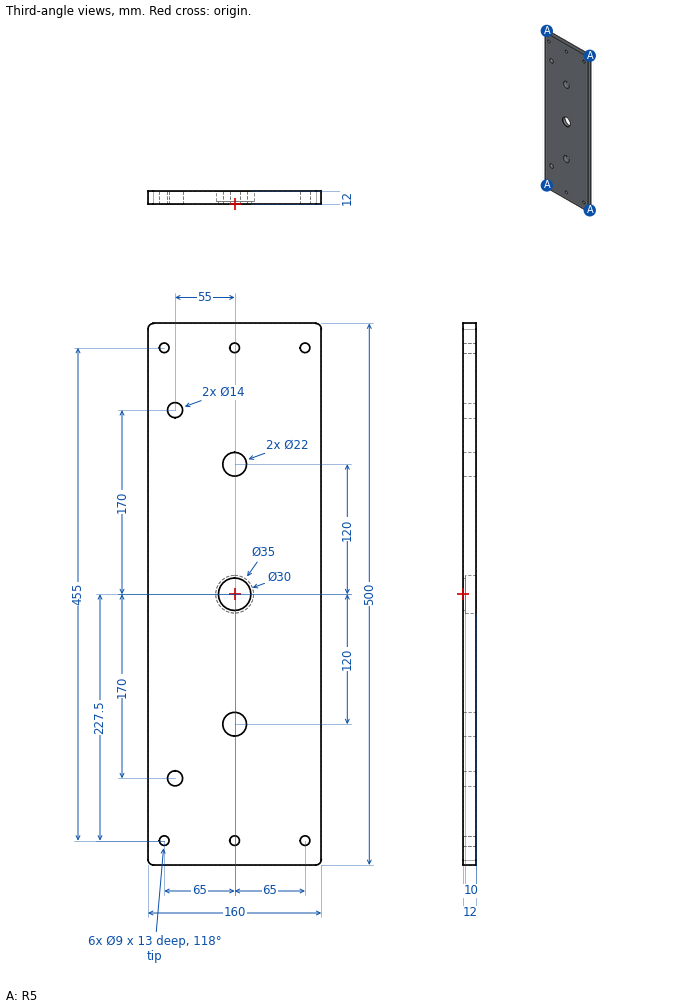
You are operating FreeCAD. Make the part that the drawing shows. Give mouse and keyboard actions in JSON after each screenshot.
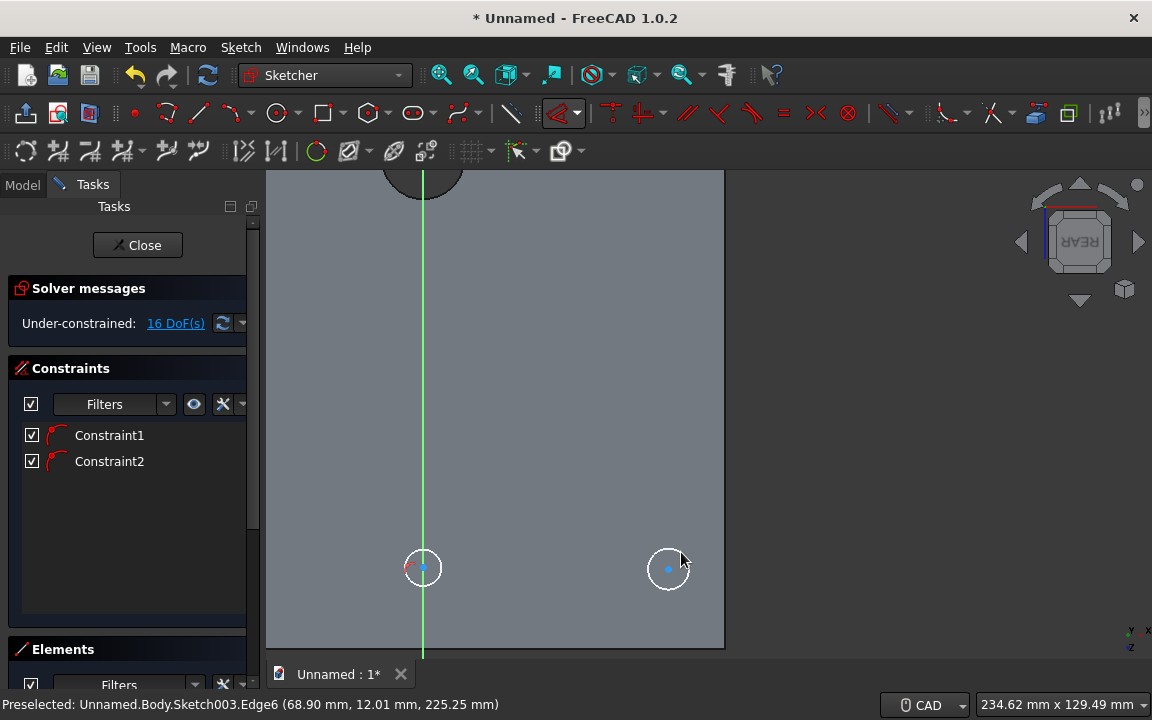
{"action": "scroll", "coordinate": [684, 555], "scroll_direction": "down", "scroll_amount": 9}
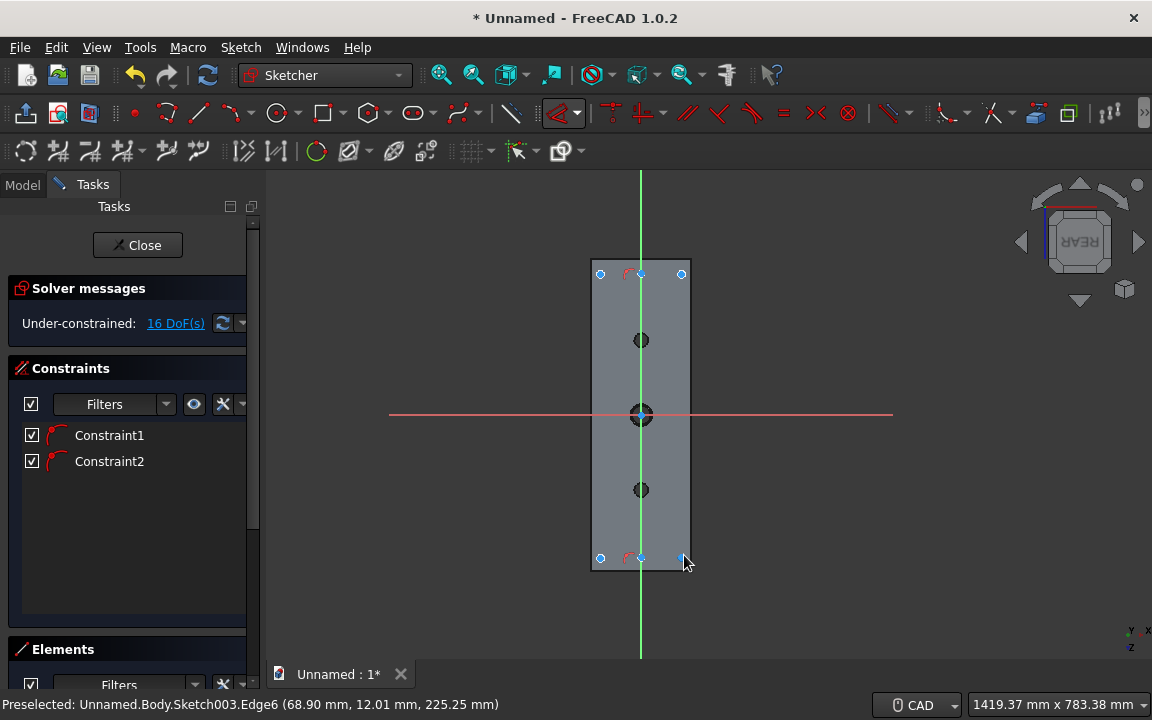
{"action": "scroll", "coordinate": [603, 272], "scroll_direction": "up", "scroll_amount": 7}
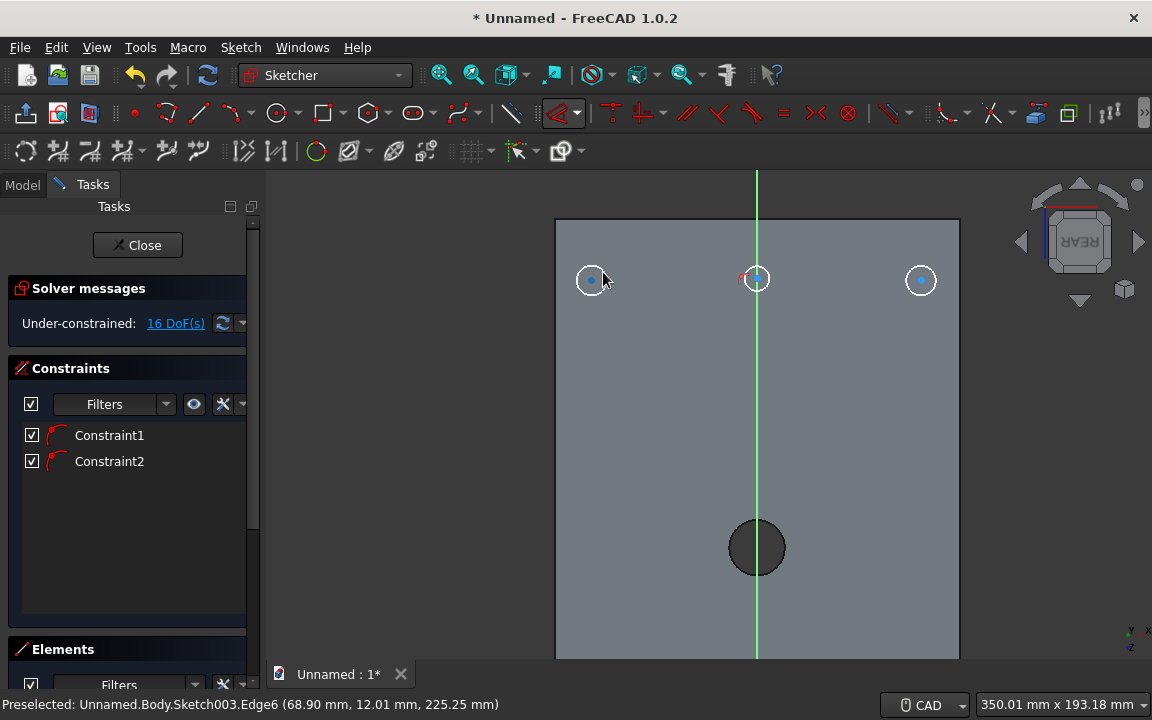
{"action": "left_click", "coordinate": [602, 270]}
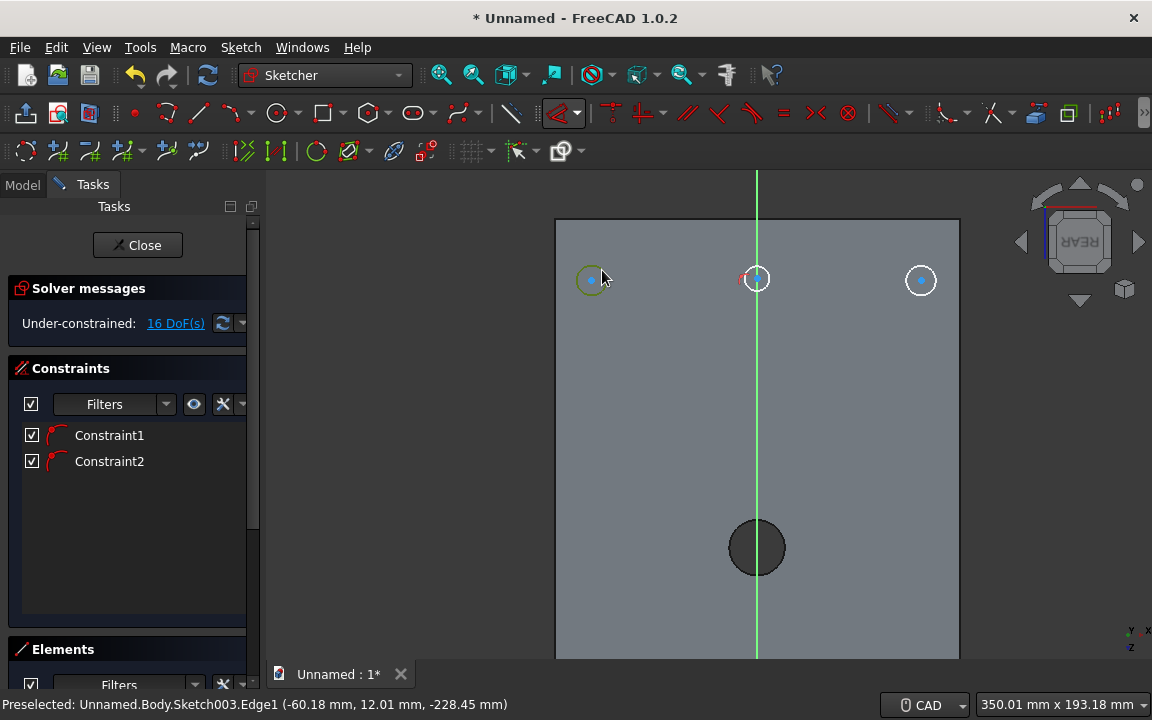
{"action": "left_click", "coordinate": [757, 266]}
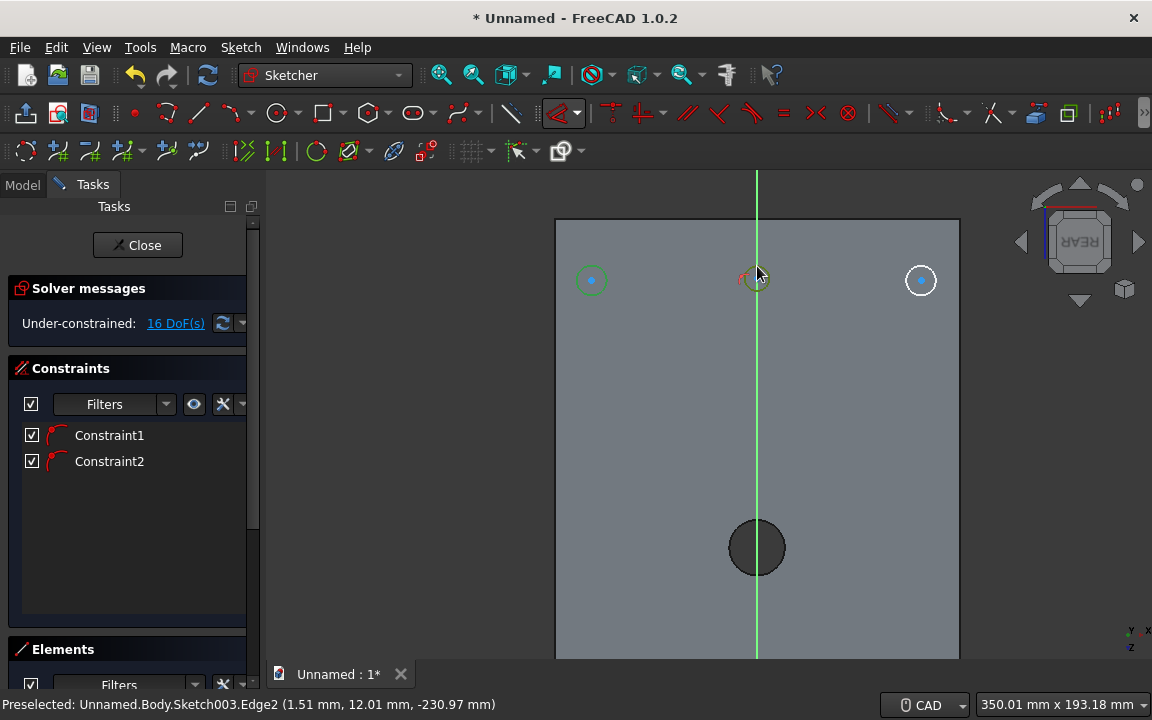
{"action": "left_click", "coordinate": [931, 270]}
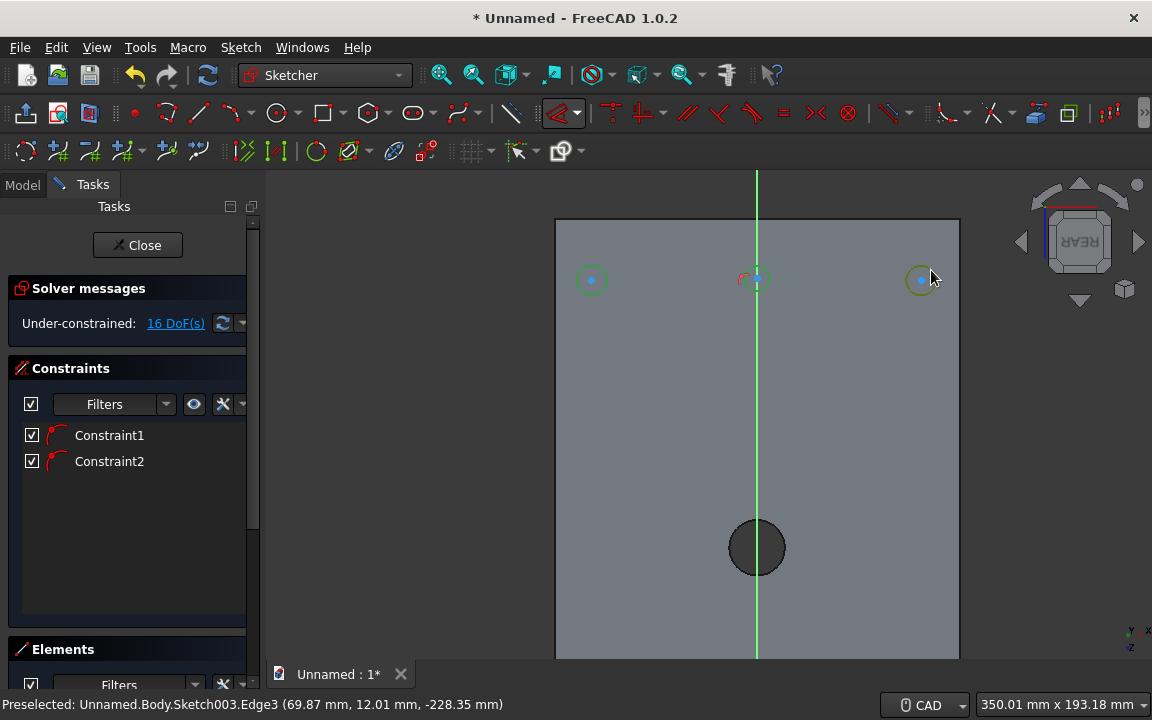
{"action": "scroll", "coordinate": [602, 271], "scroll_direction": "down", "scroll_amount": 7}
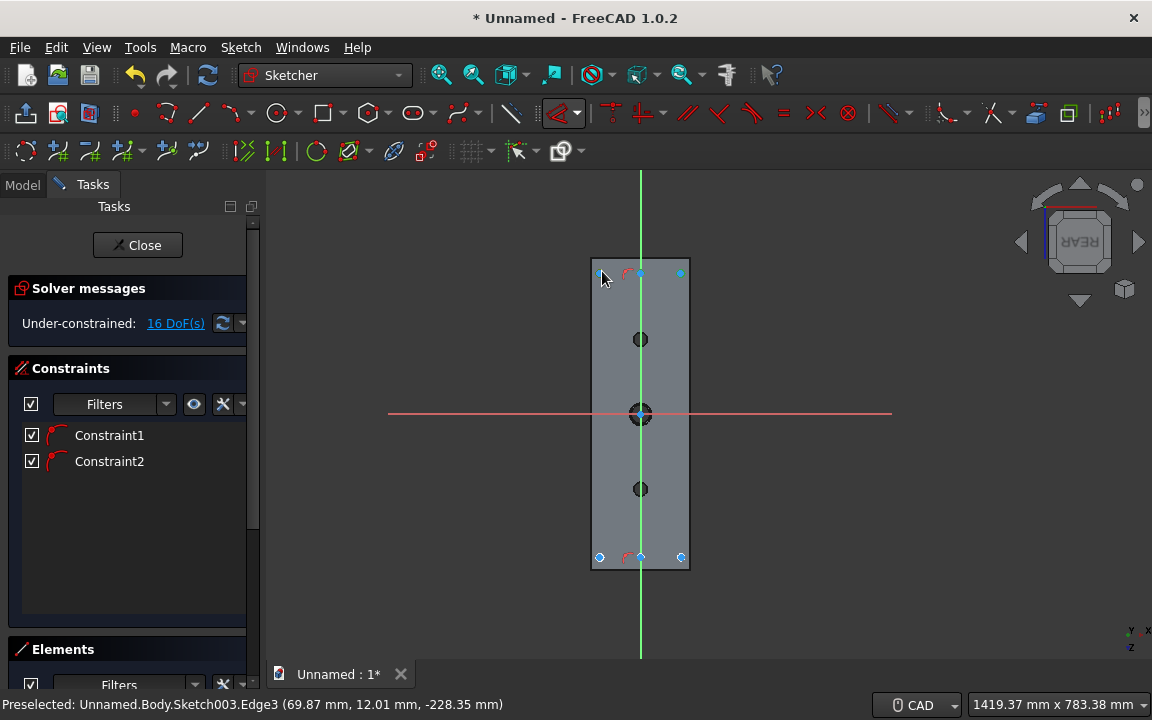
{"action": "scroll", "coordinate": [603, 555], "scroll_direction": "up", "scroll_amount": 7}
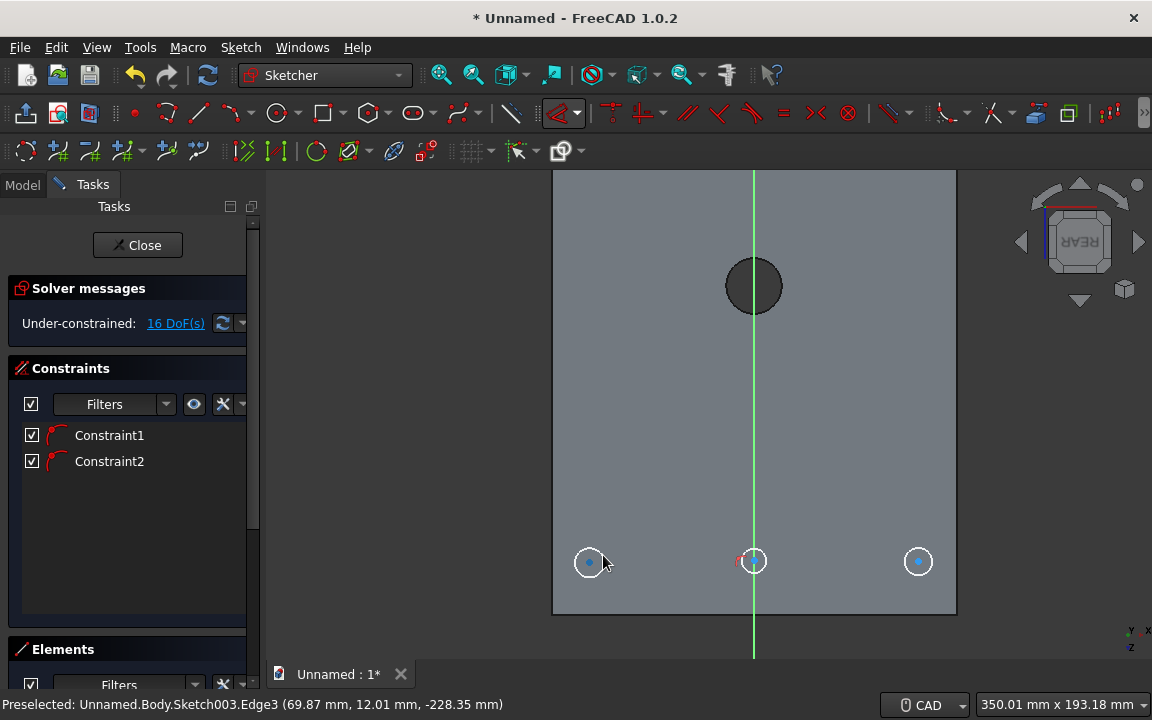
{"action": "left_click", "coordinate": [600, 553]}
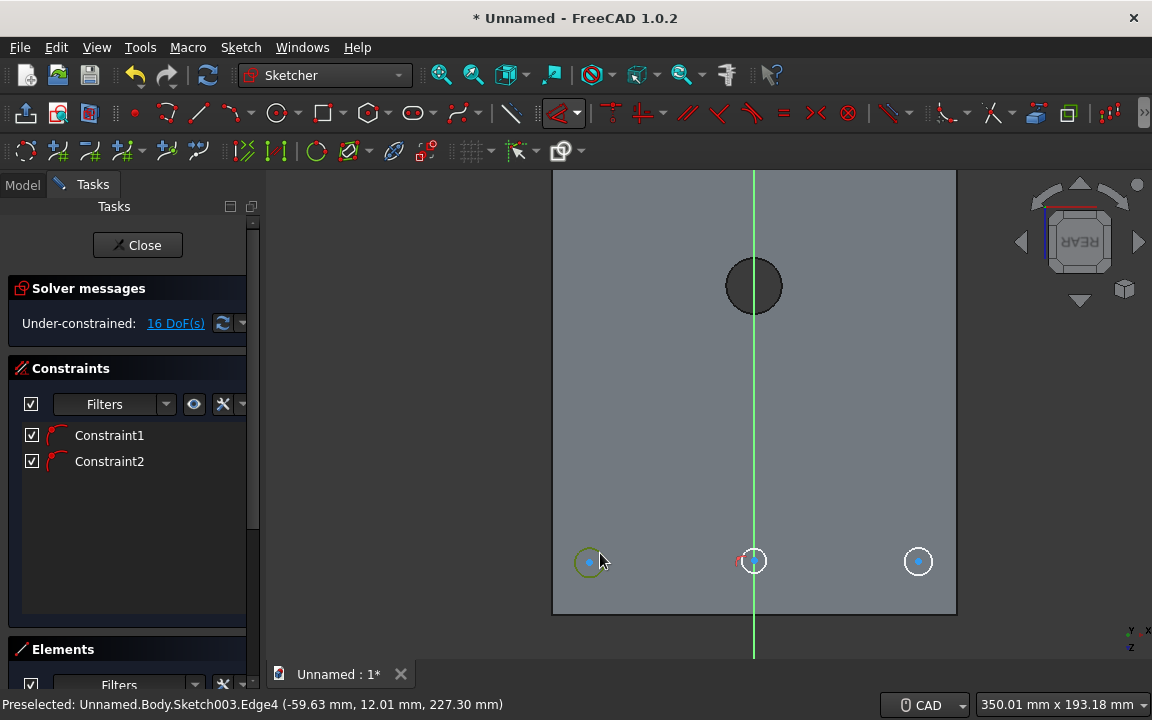
{"action": "left_click", "coordinate": [754, 549]}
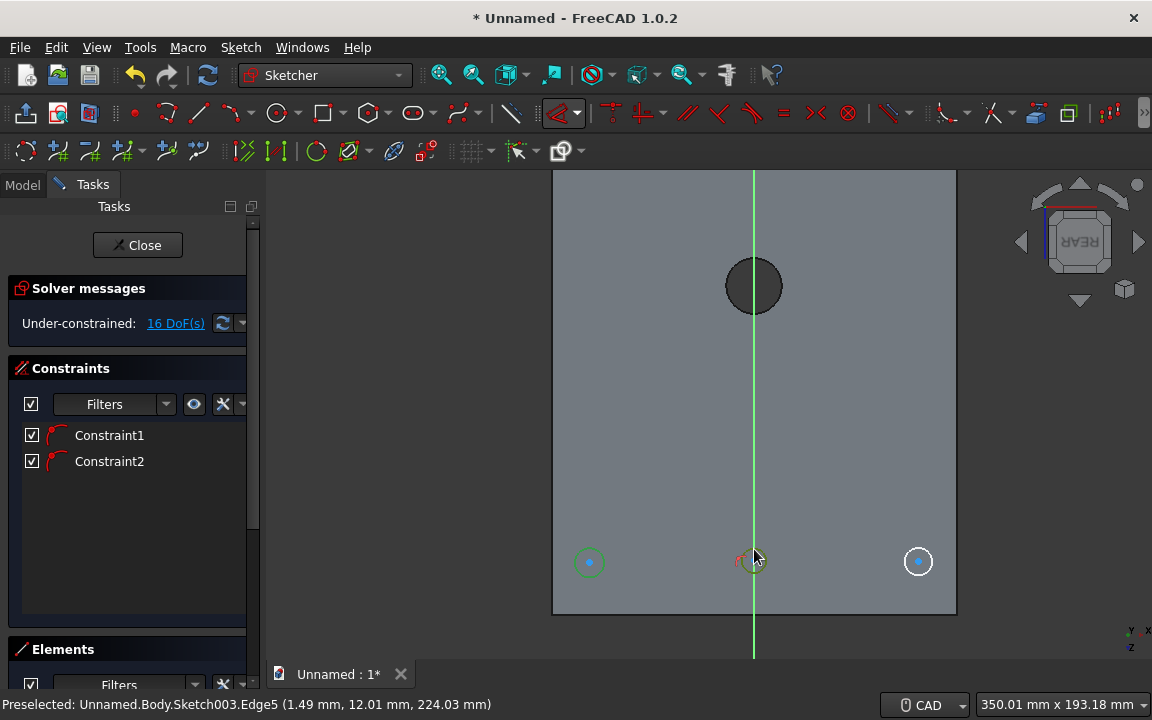
{"action": "left_click", "coordinate": [928, 552]}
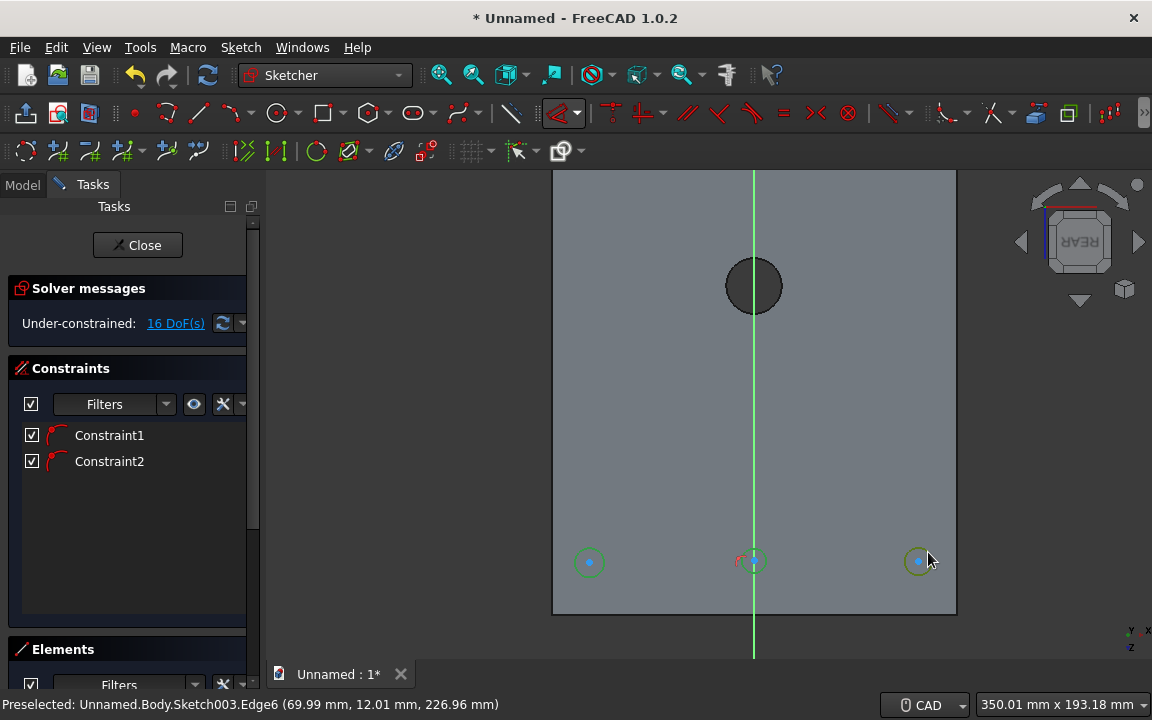
{"action": "left_click", "coordinate": [784, 114]}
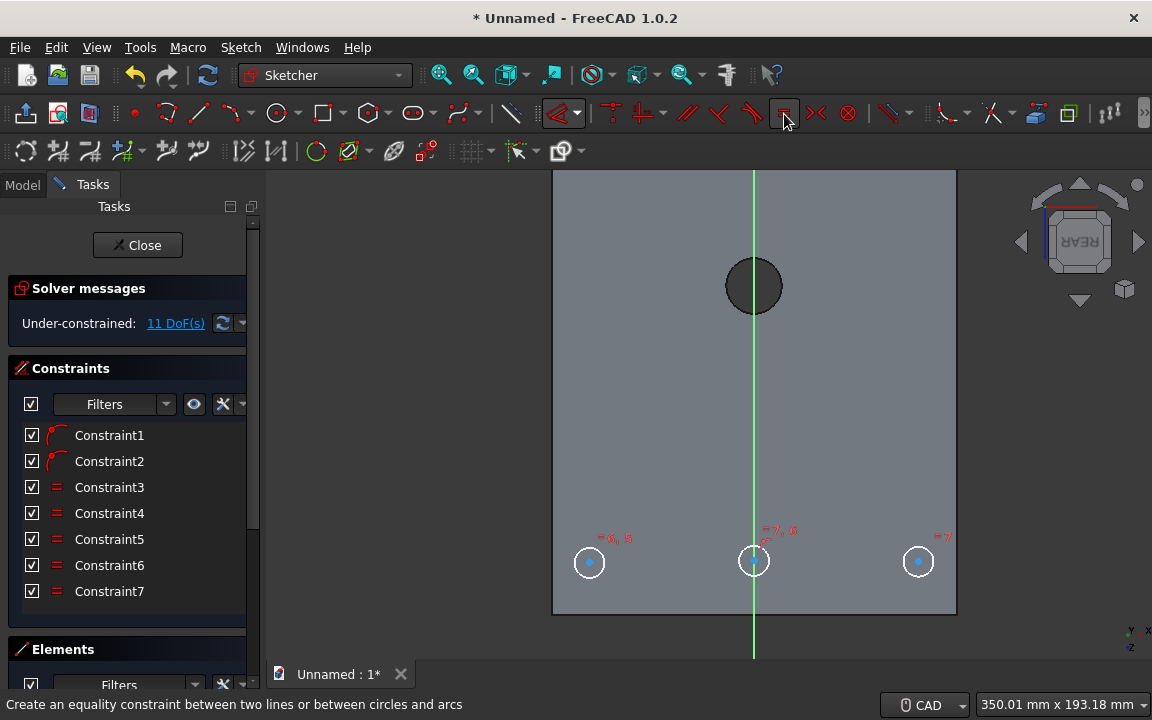
{"action": "scroll", "coordinate": [603, 556], "scroll_direction": "down", "scroll_amount": 7}